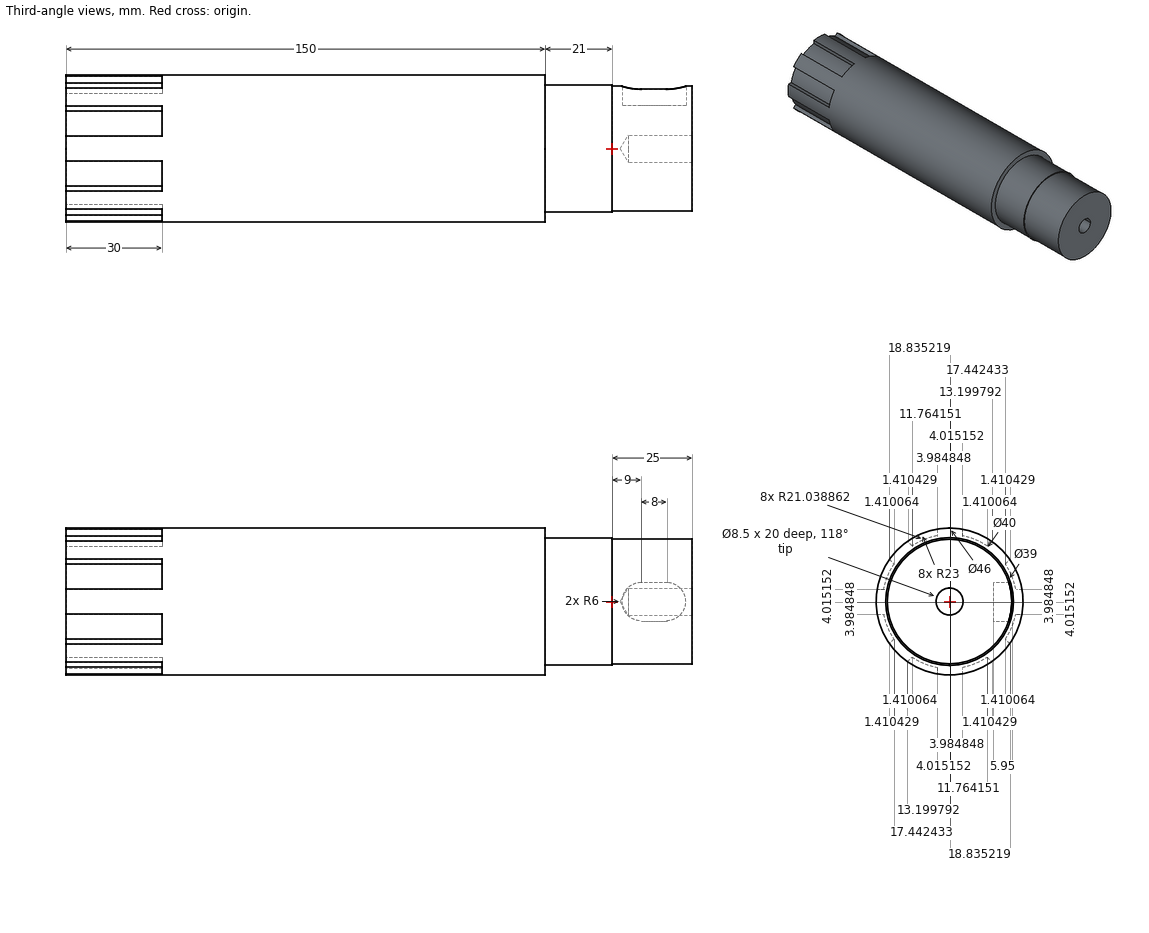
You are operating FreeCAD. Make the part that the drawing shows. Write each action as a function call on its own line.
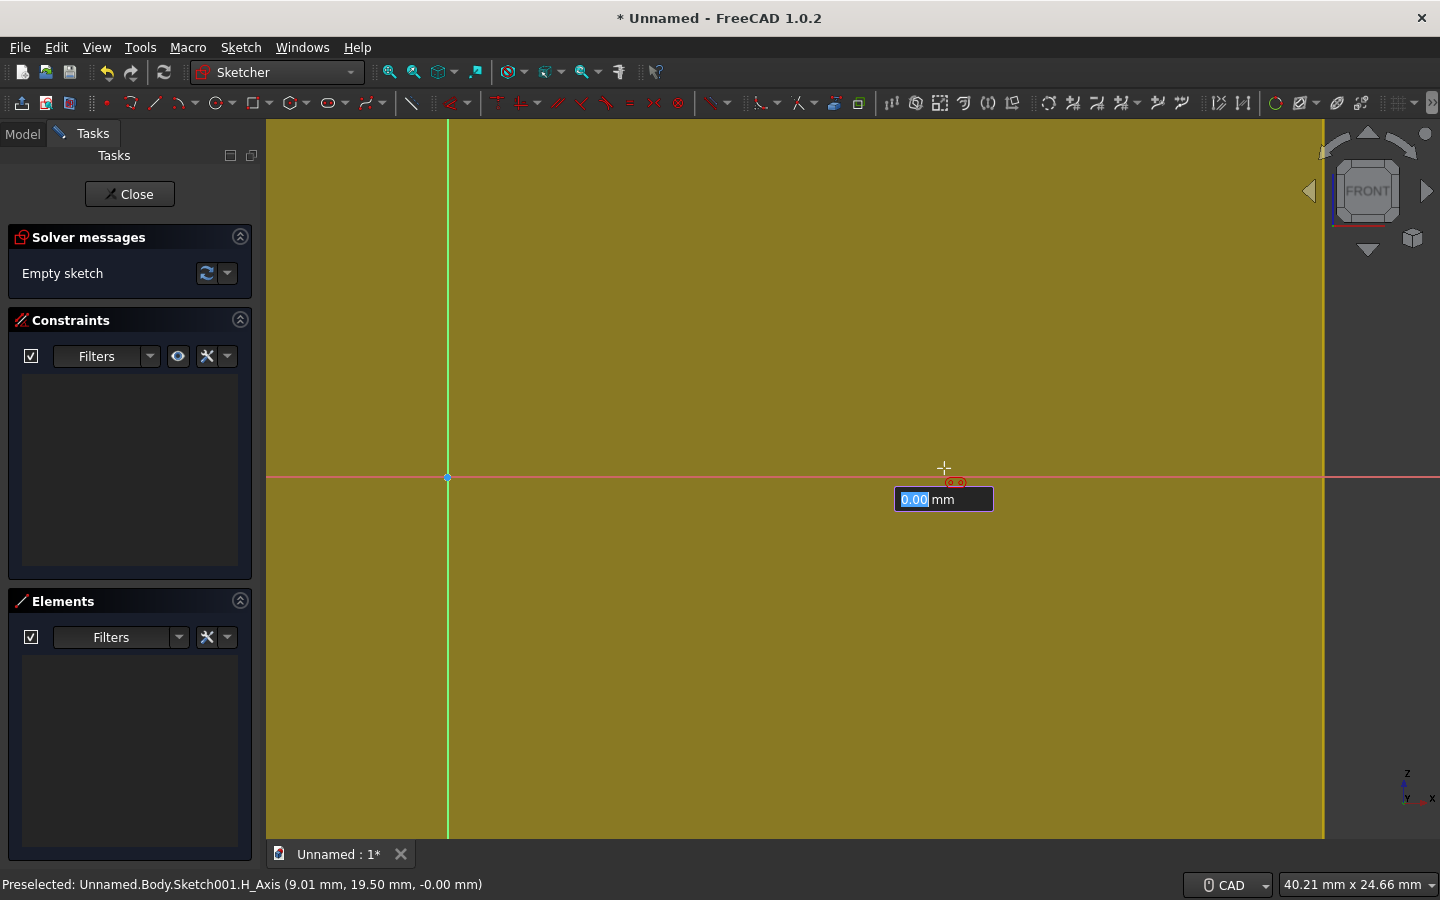
click(827, 653)
key(Escape)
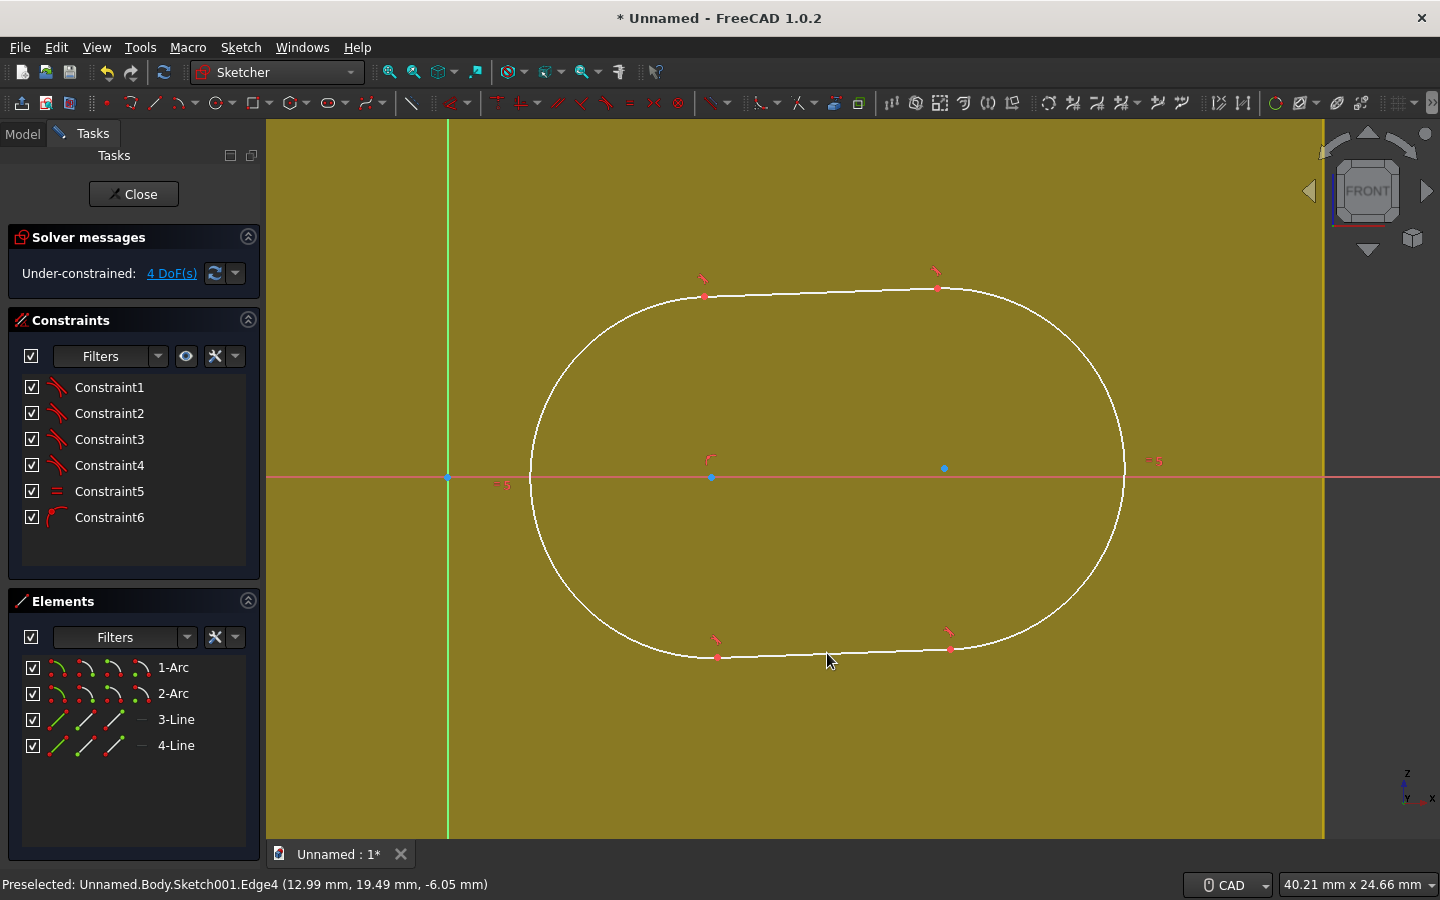
click(774, 294)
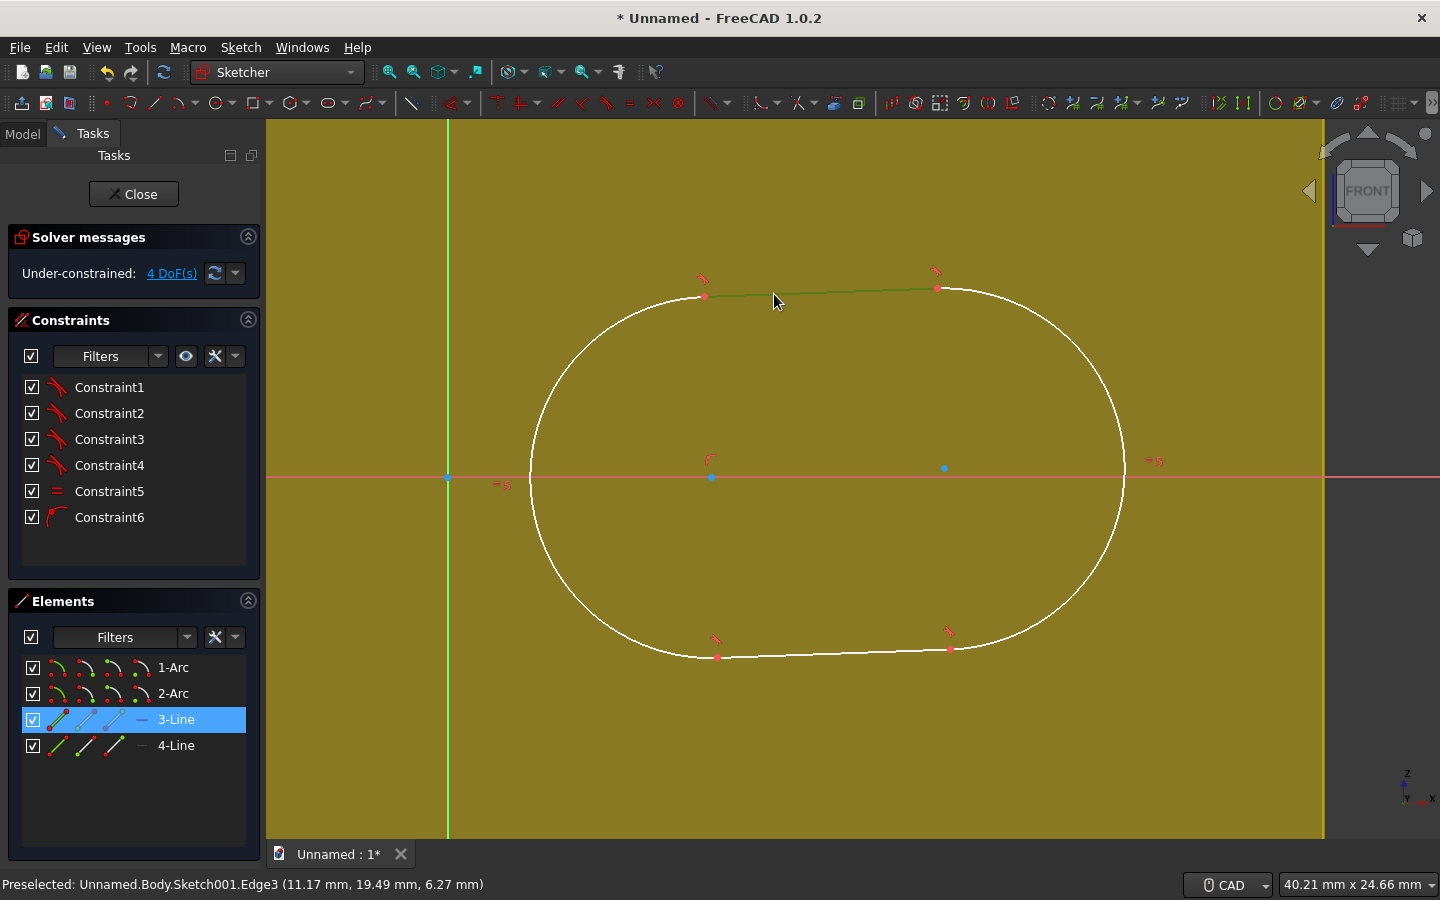
key(h)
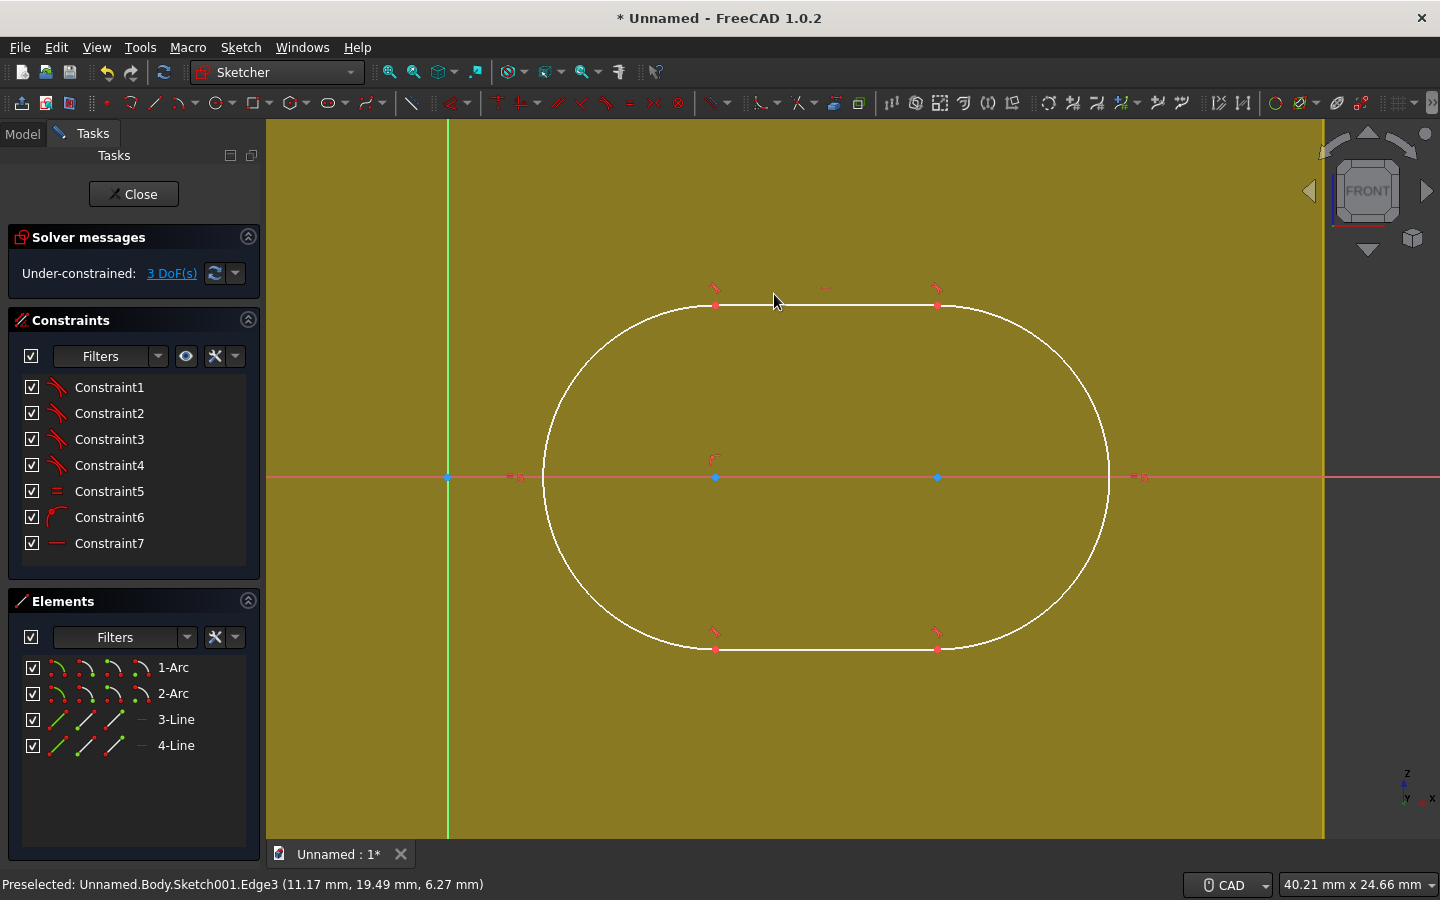
click(450, 104)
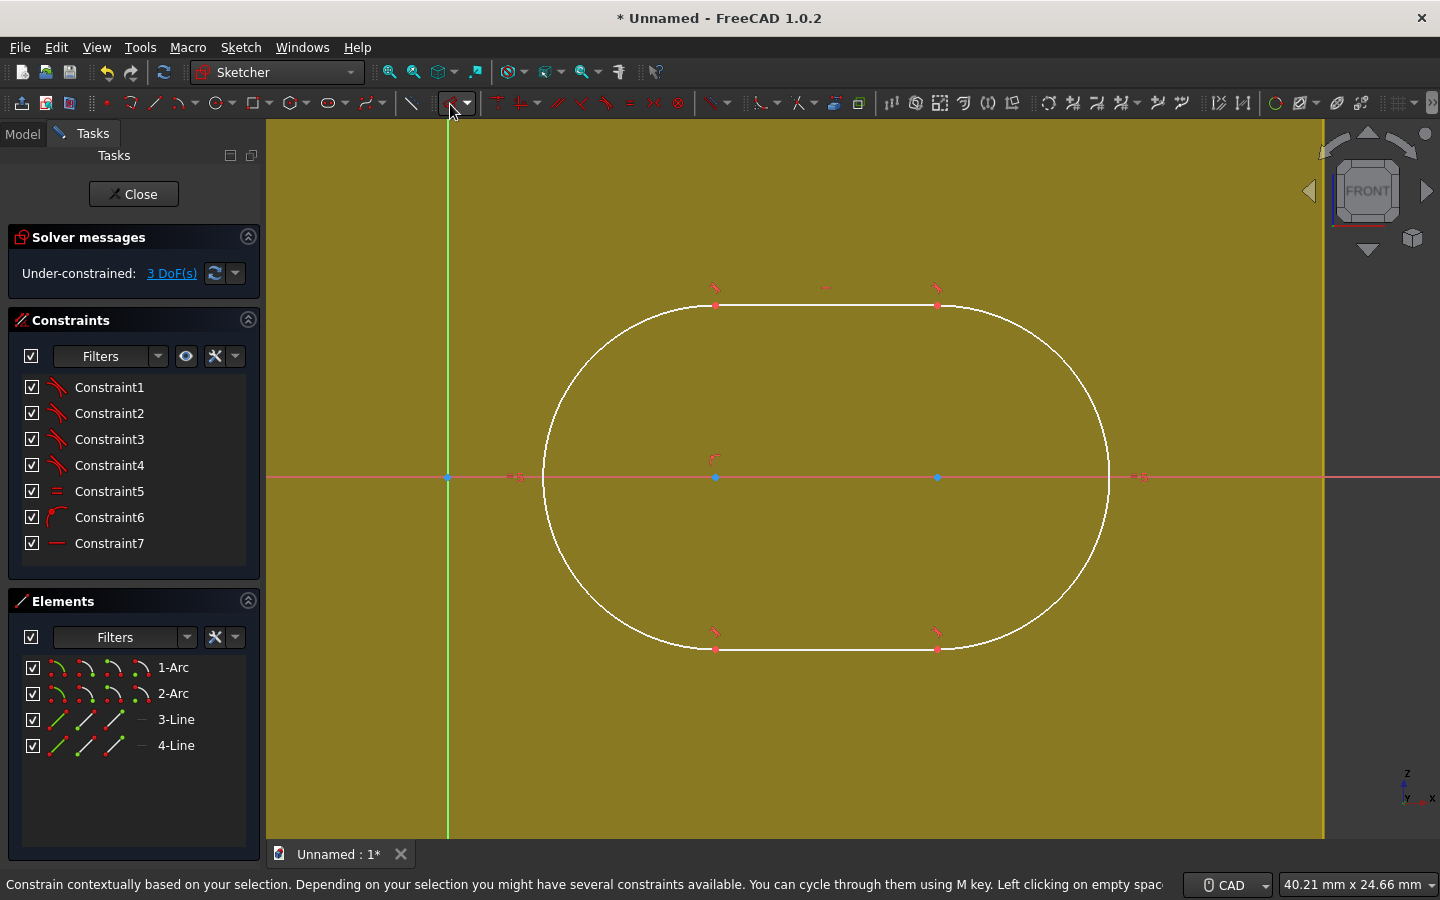
click(576, 376)
click(550, 357)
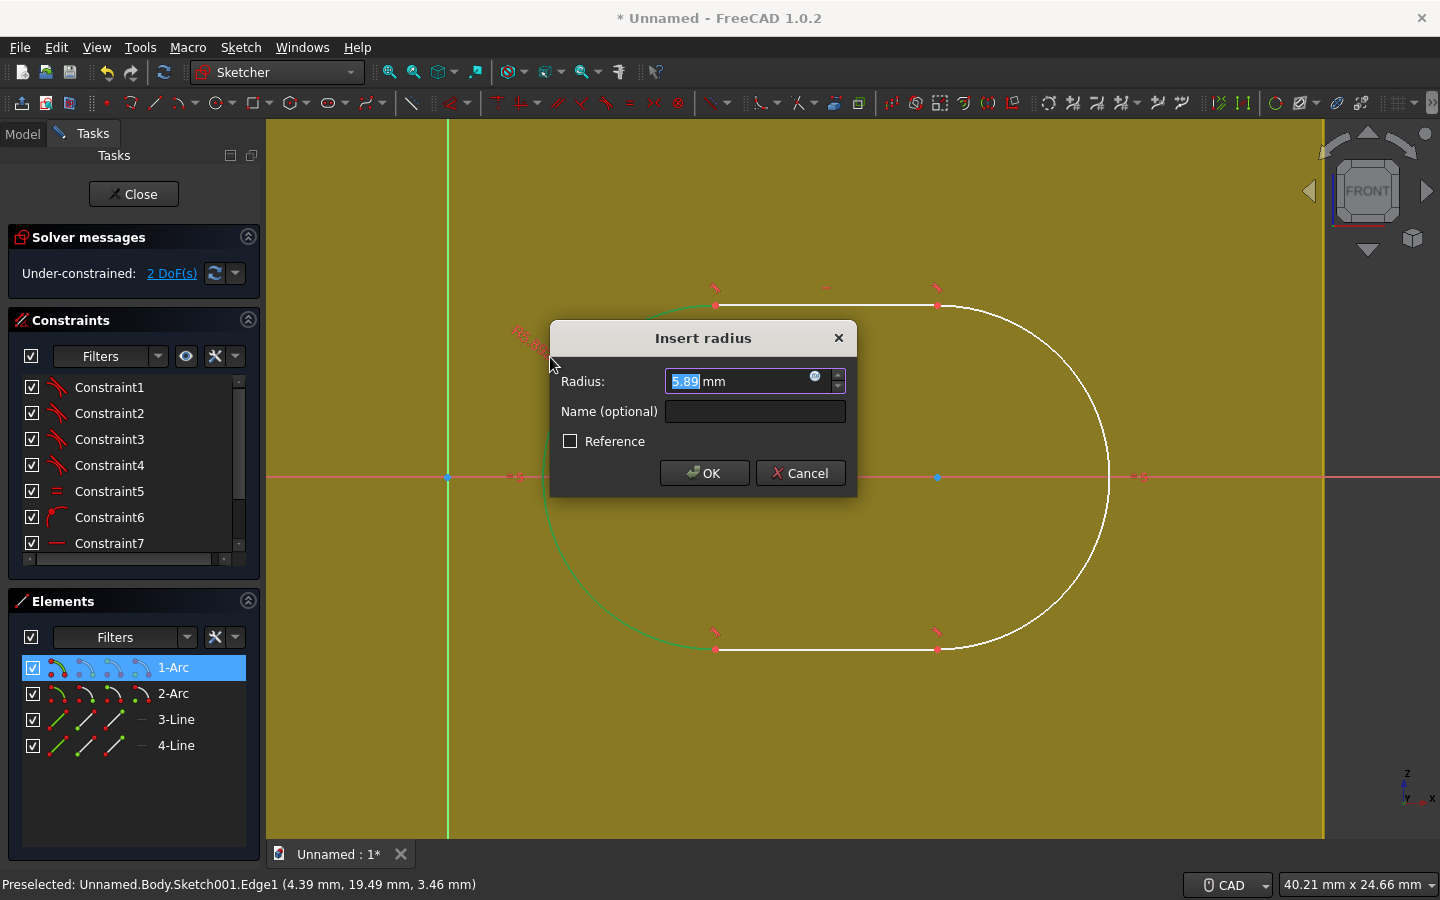
text(6)
key(Return)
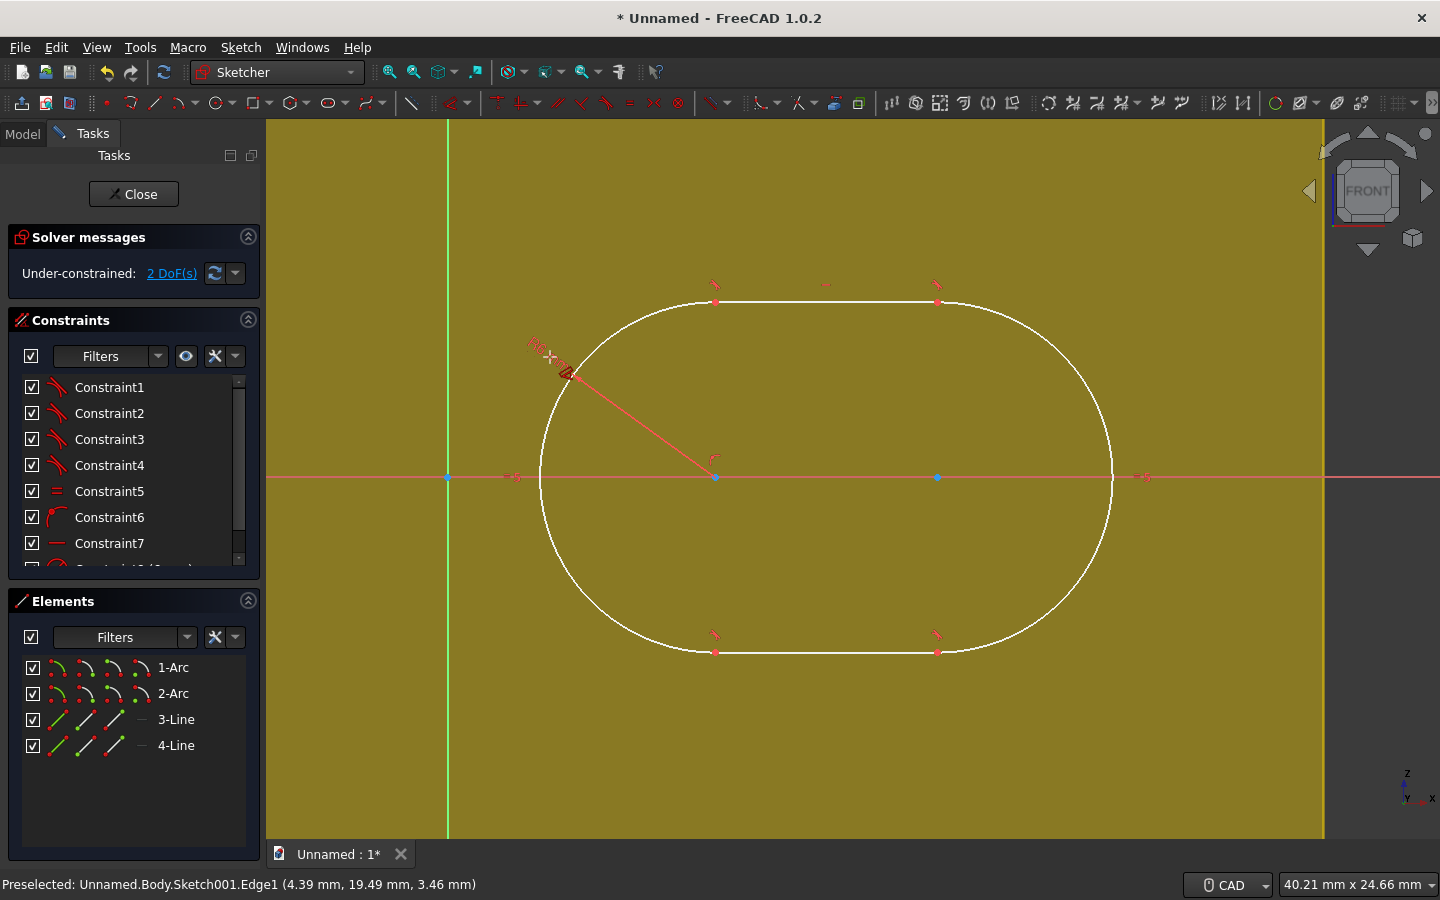
click(782, 302)
click(826, 268)